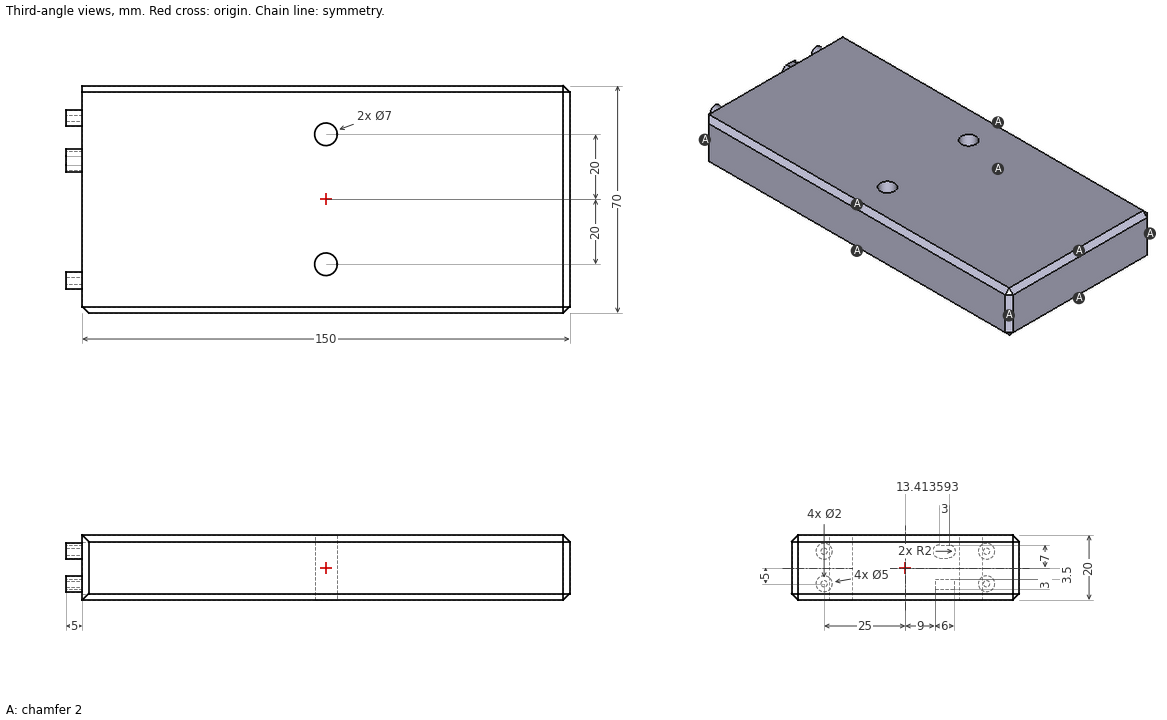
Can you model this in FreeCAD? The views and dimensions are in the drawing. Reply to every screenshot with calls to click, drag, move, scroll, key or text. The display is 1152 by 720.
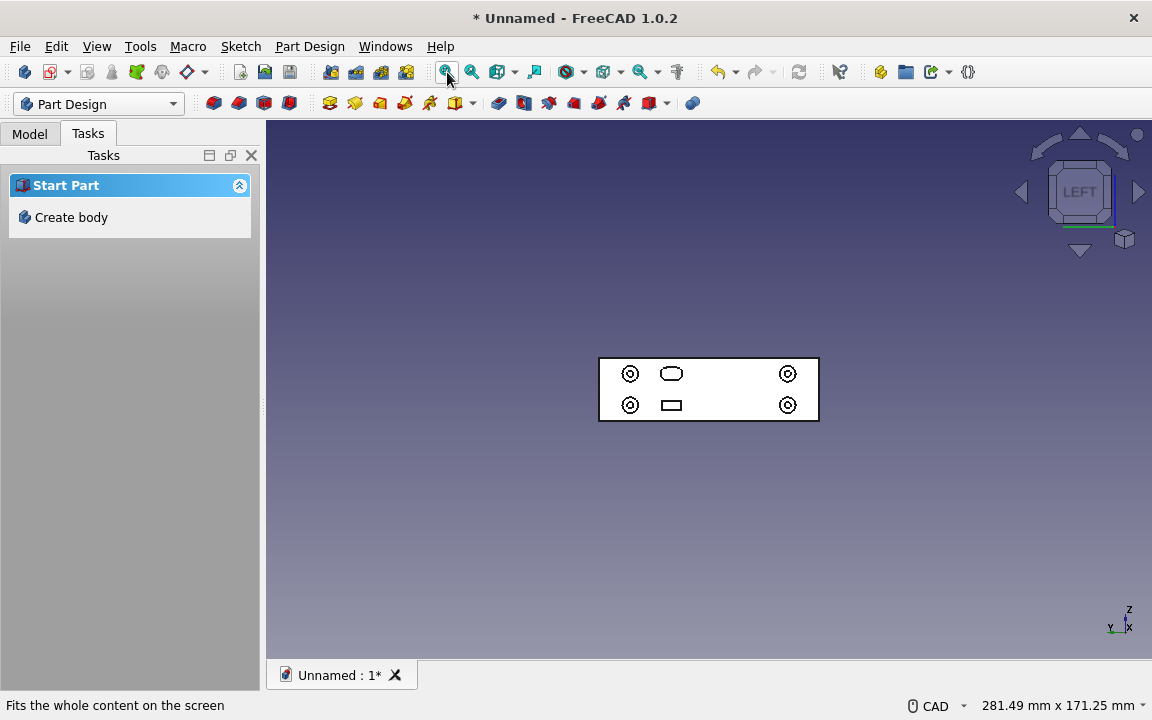
key(0)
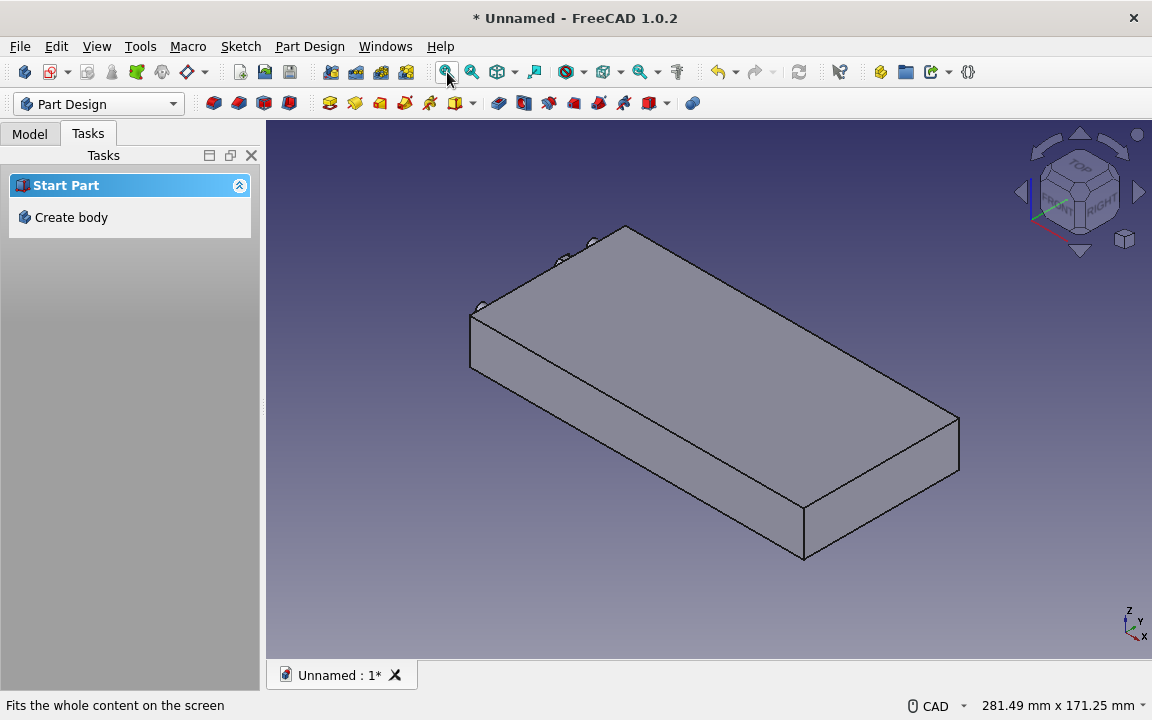
click(780, 519)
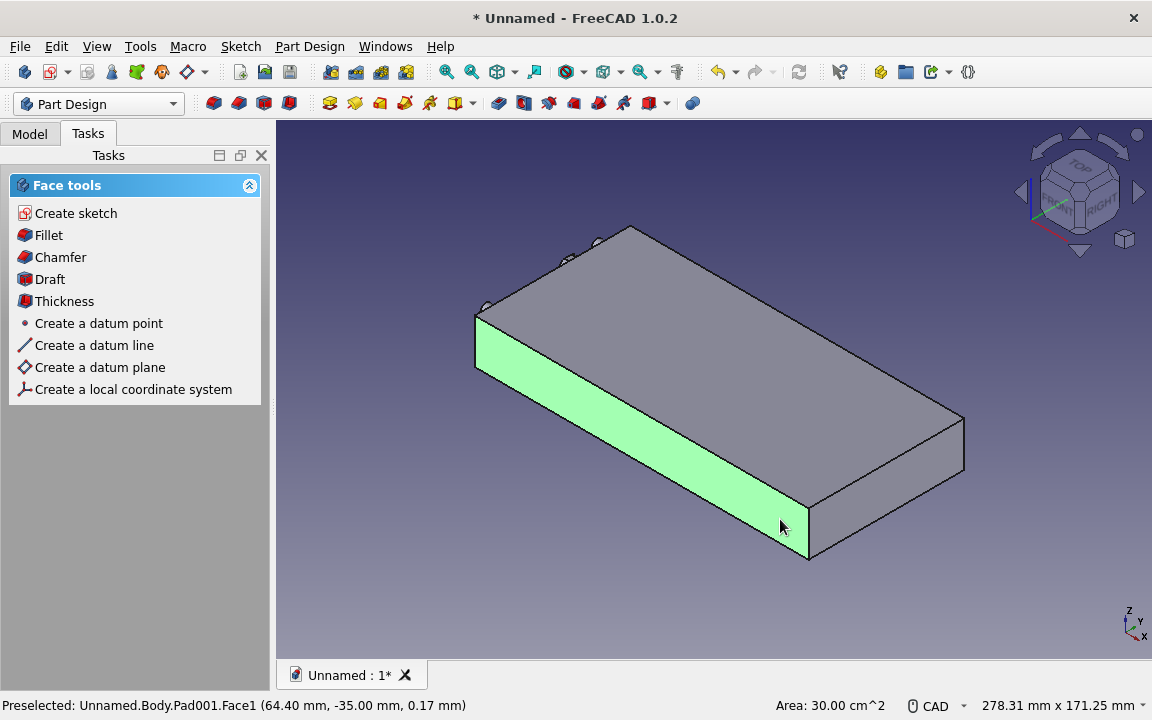
click(931, 462, ctrl)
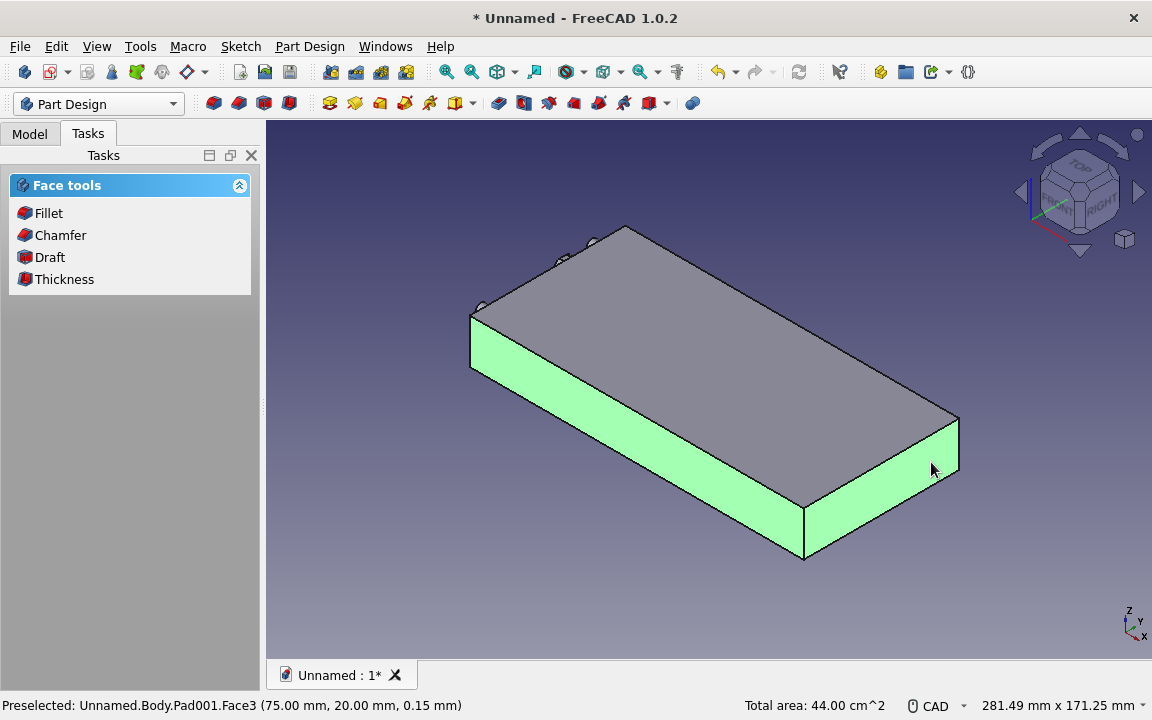
key(2)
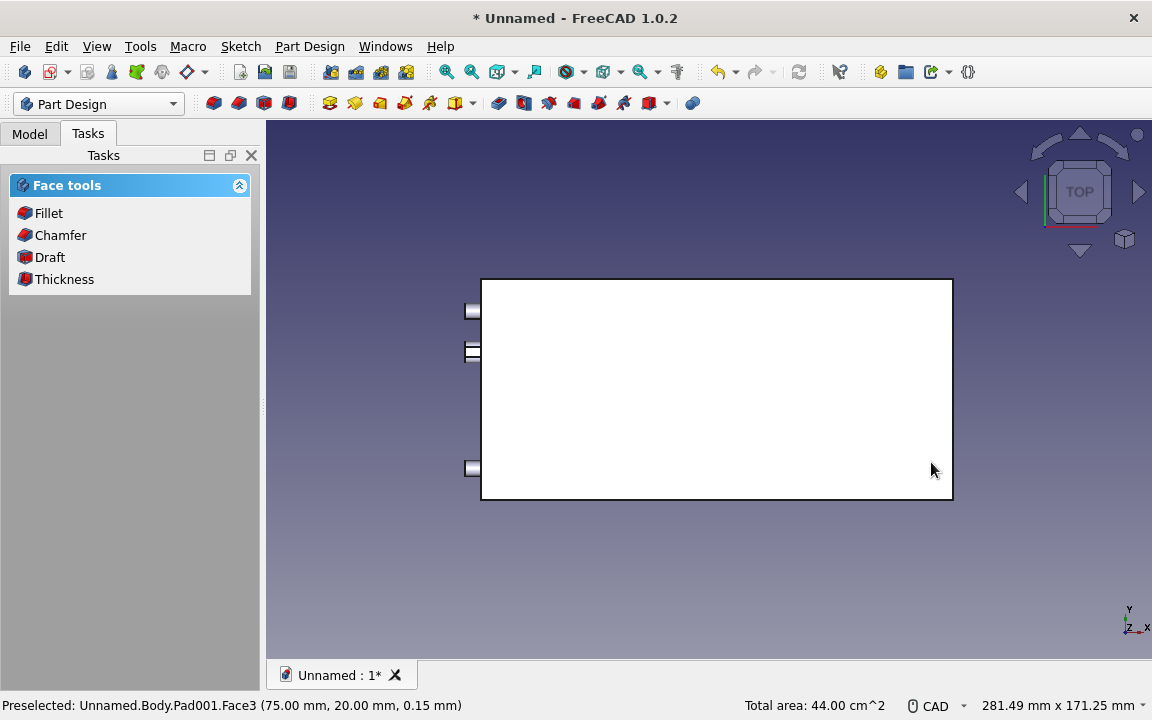
click(717, 278, ctrl)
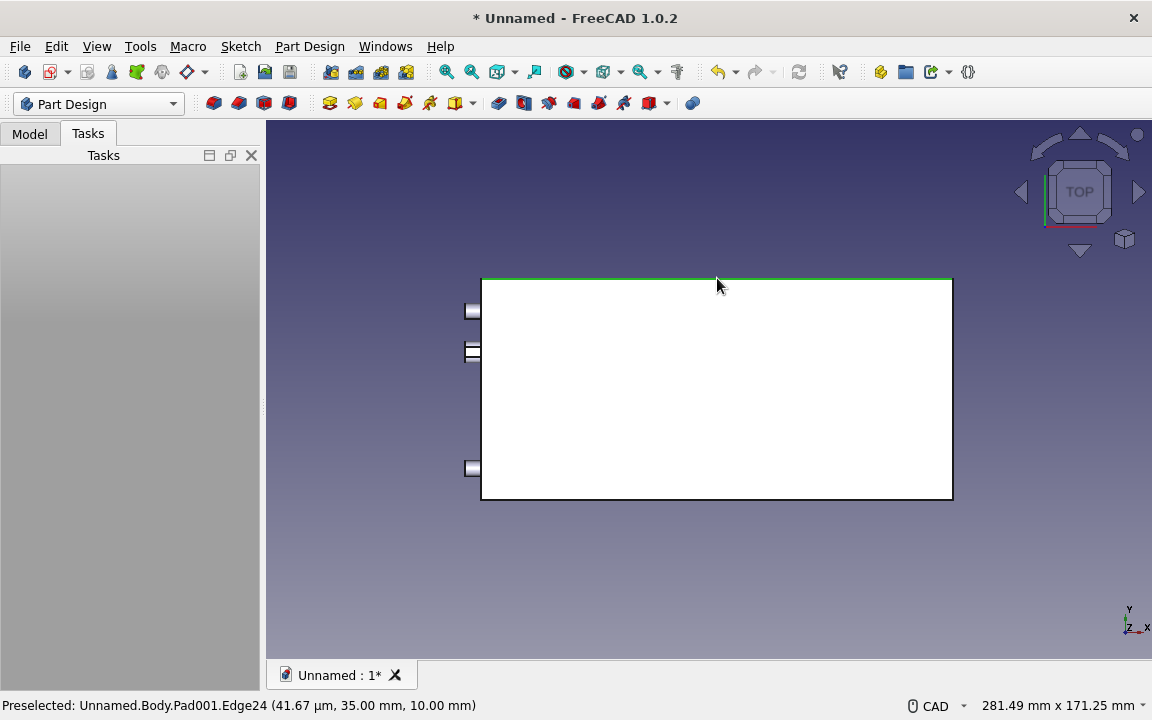
key(1)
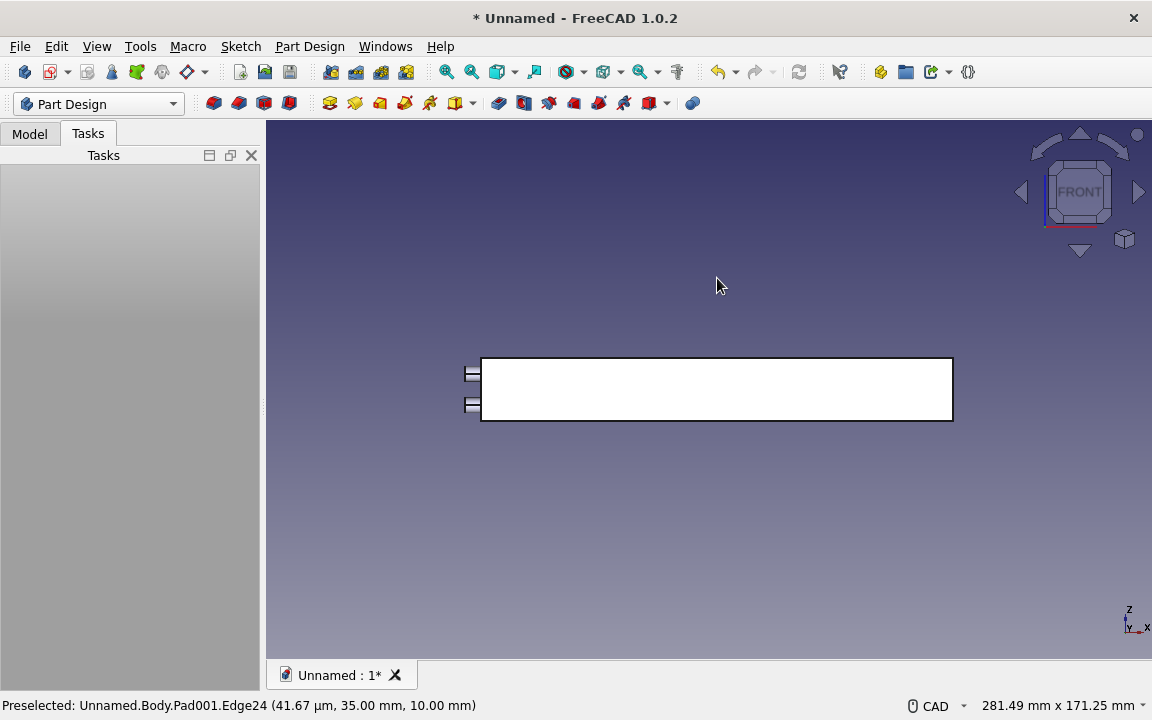
key(3)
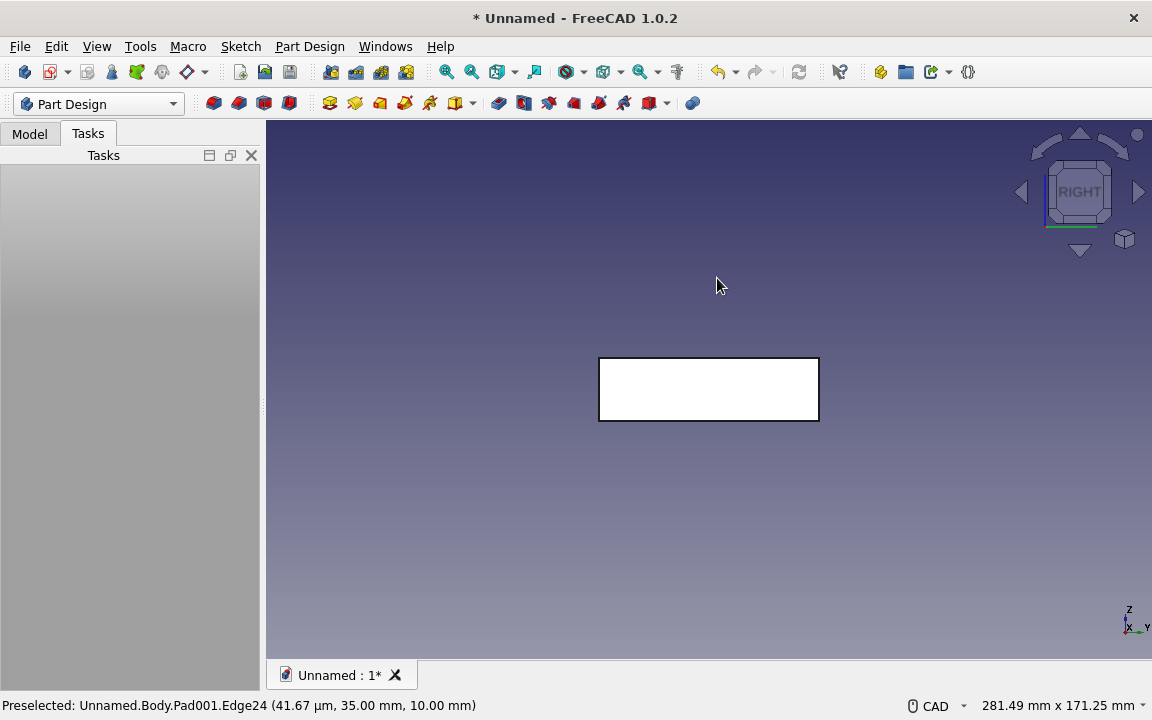
click(447, 72)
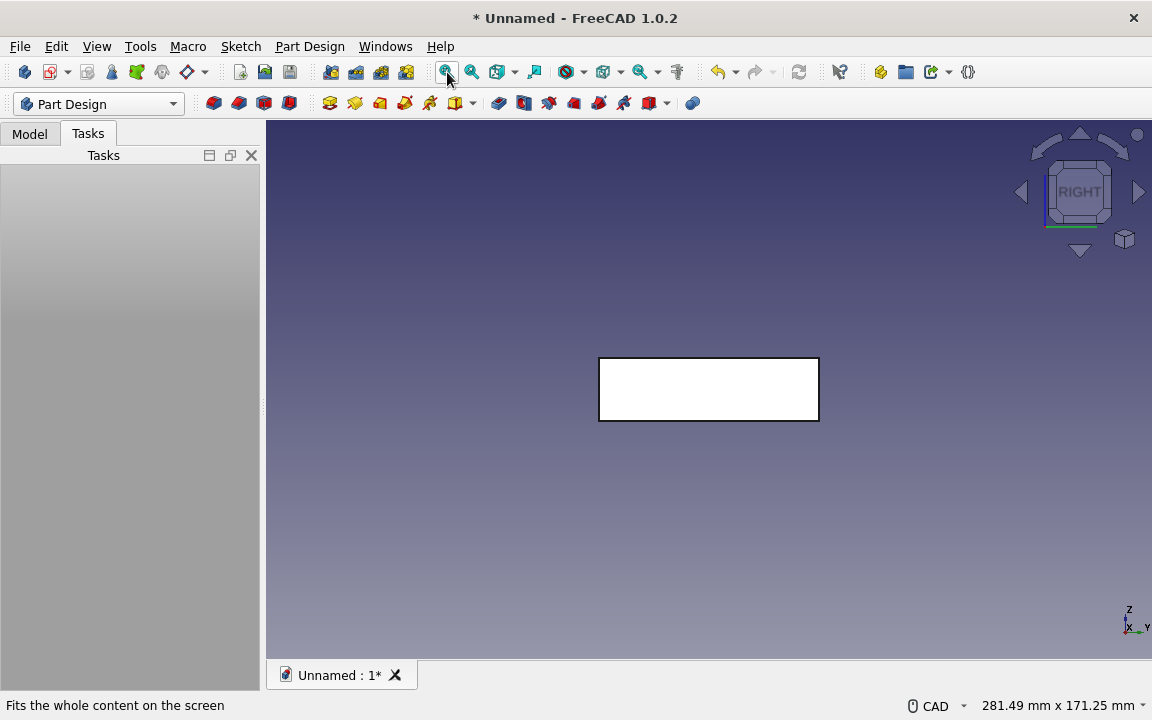
key(5)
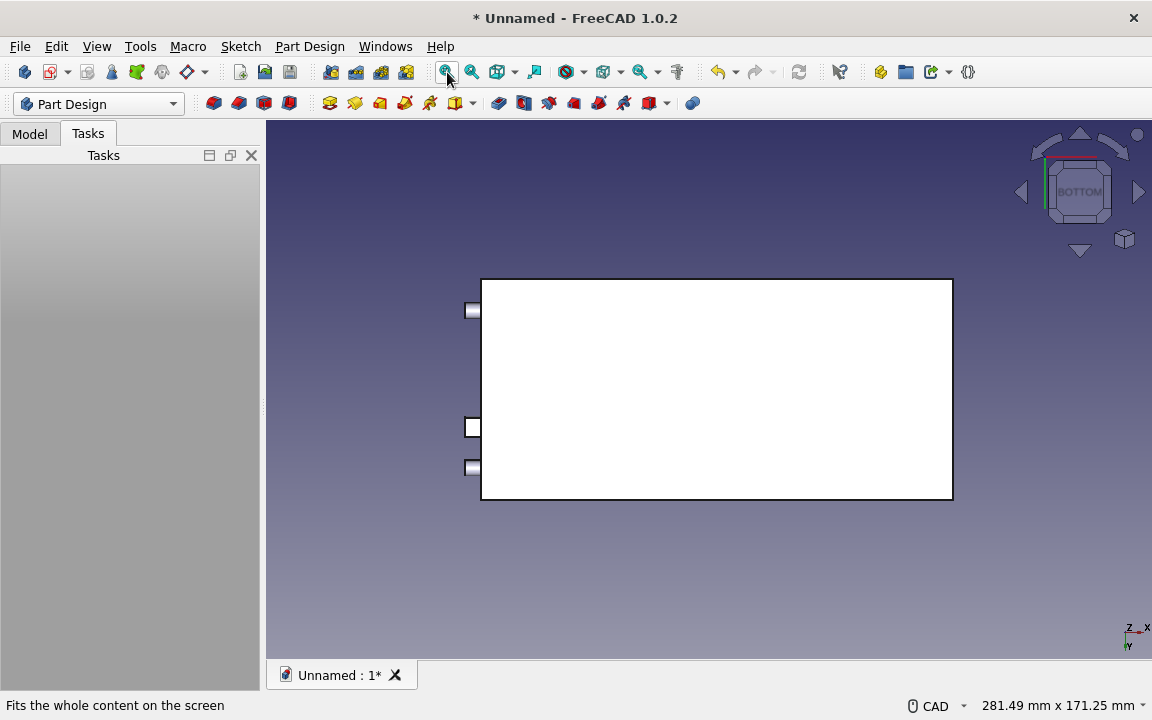
click(717, 499, ctrl)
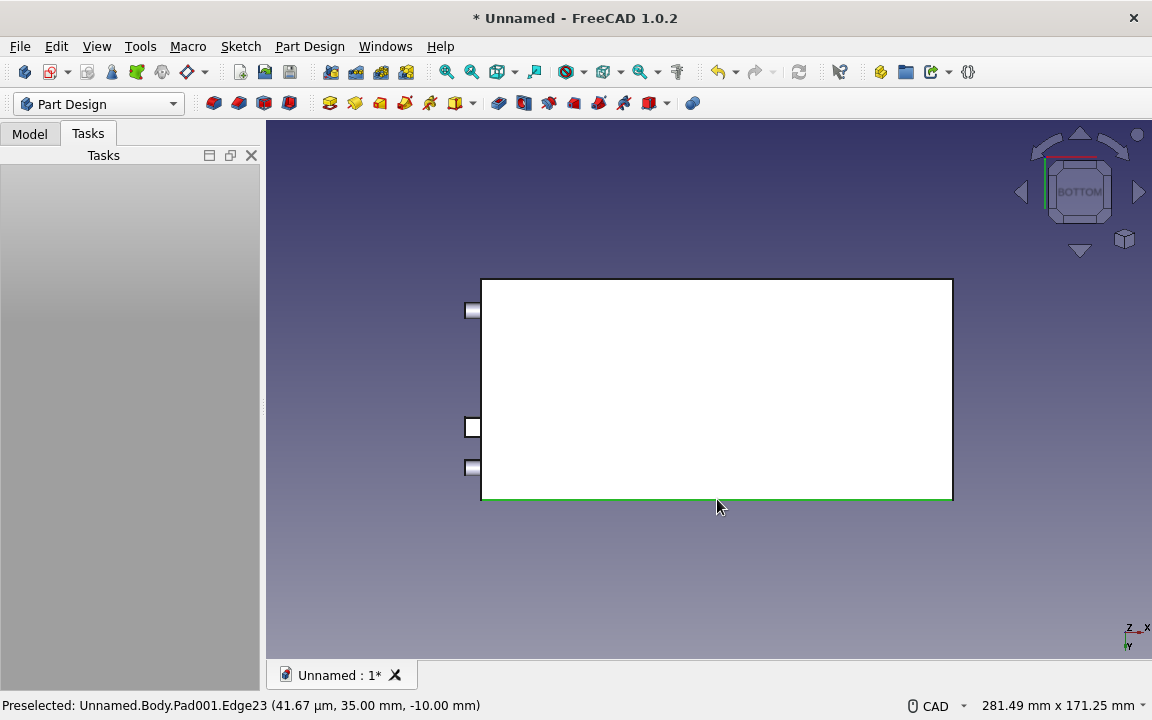
click(239, 104)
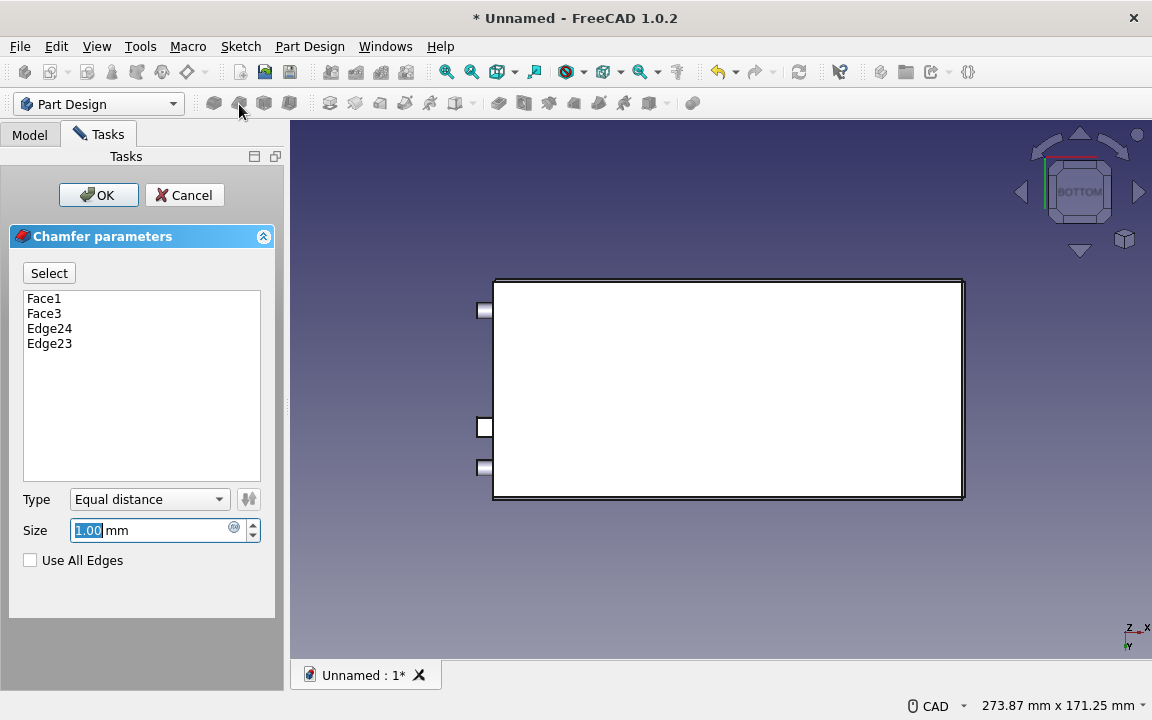
text(2)
key(Tab)